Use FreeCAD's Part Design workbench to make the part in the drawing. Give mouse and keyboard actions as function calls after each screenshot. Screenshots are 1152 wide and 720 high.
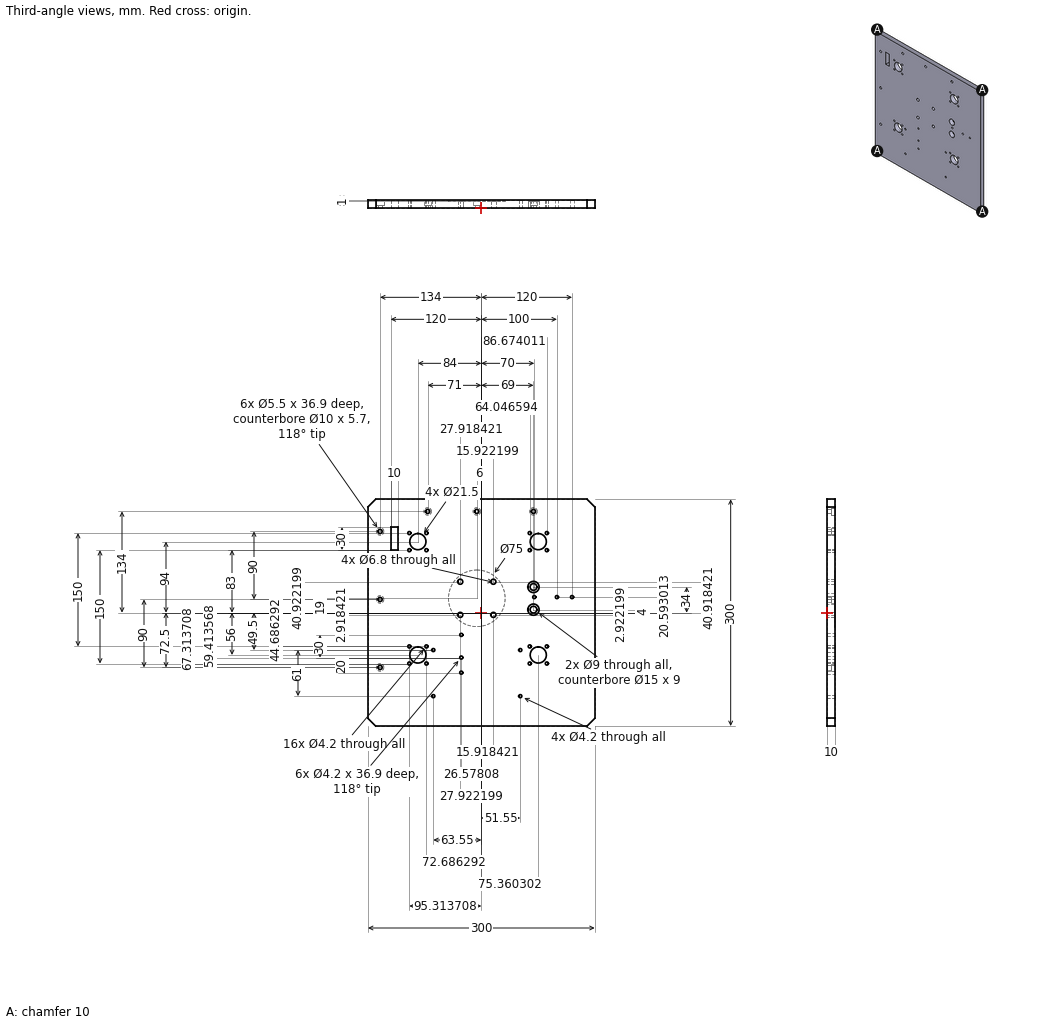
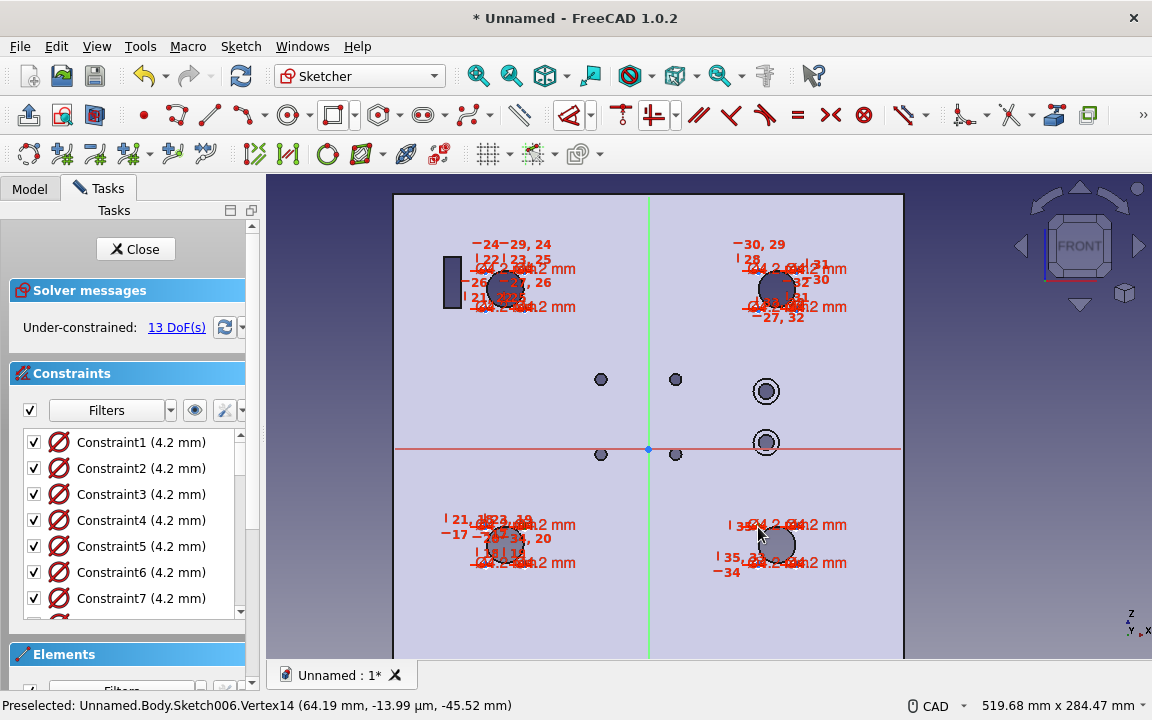
key(h)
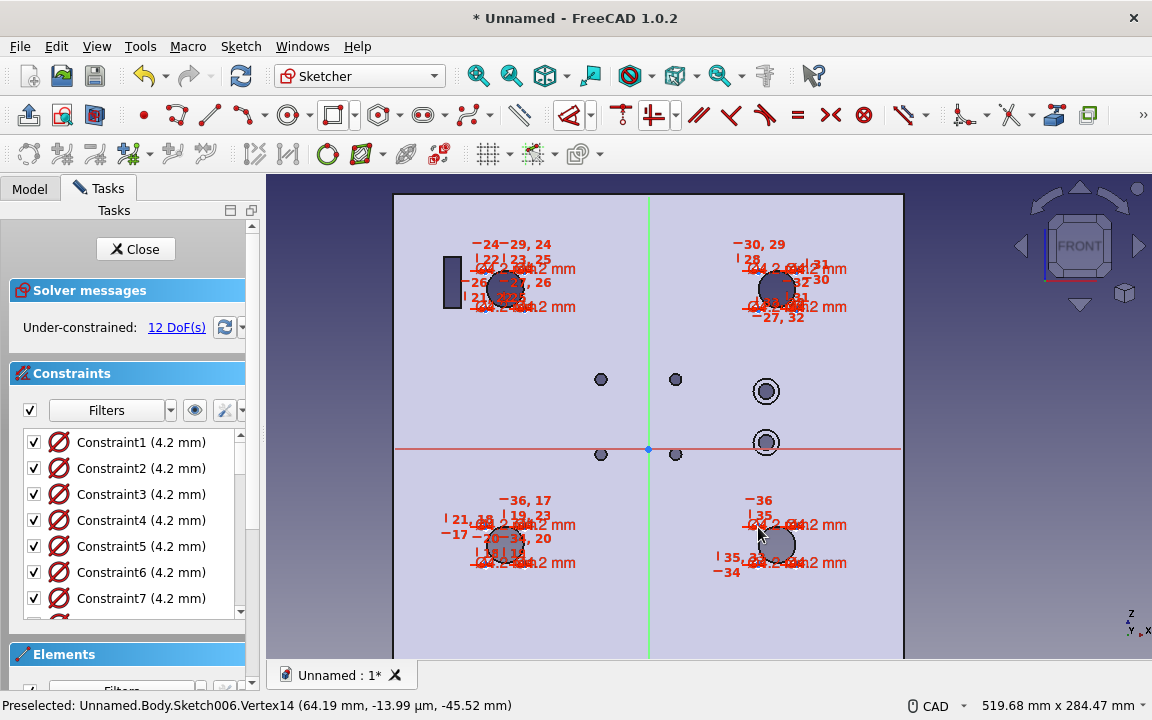
click(796, 309)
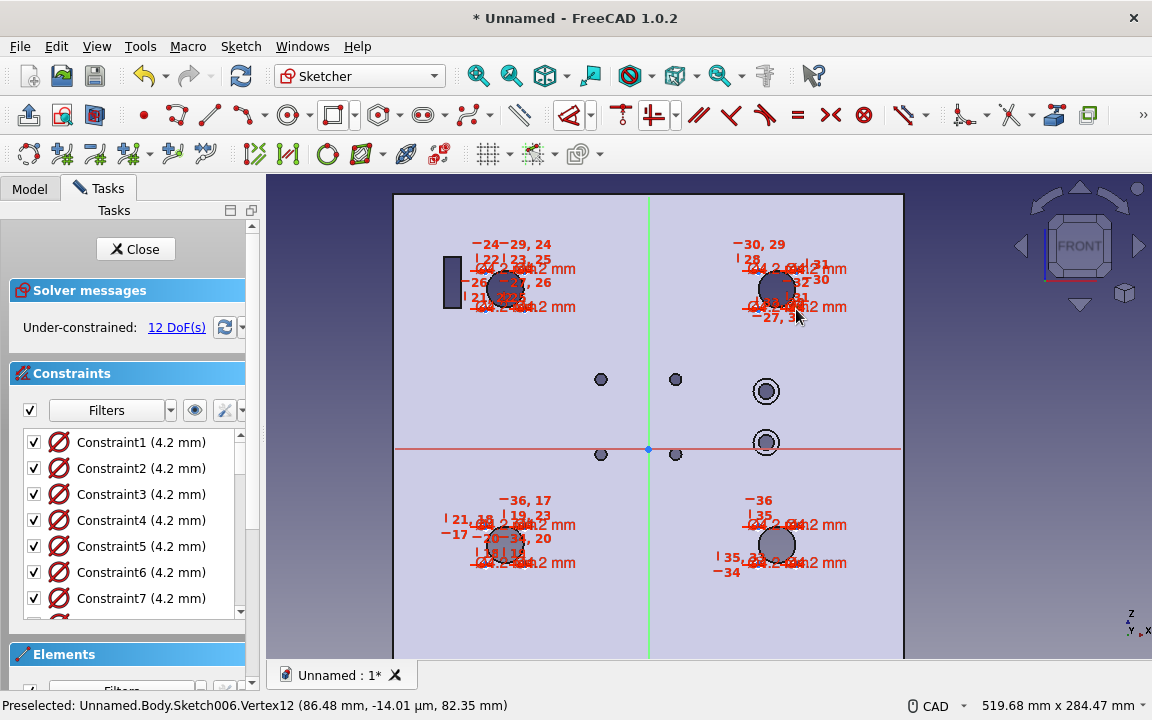
click(796, 527)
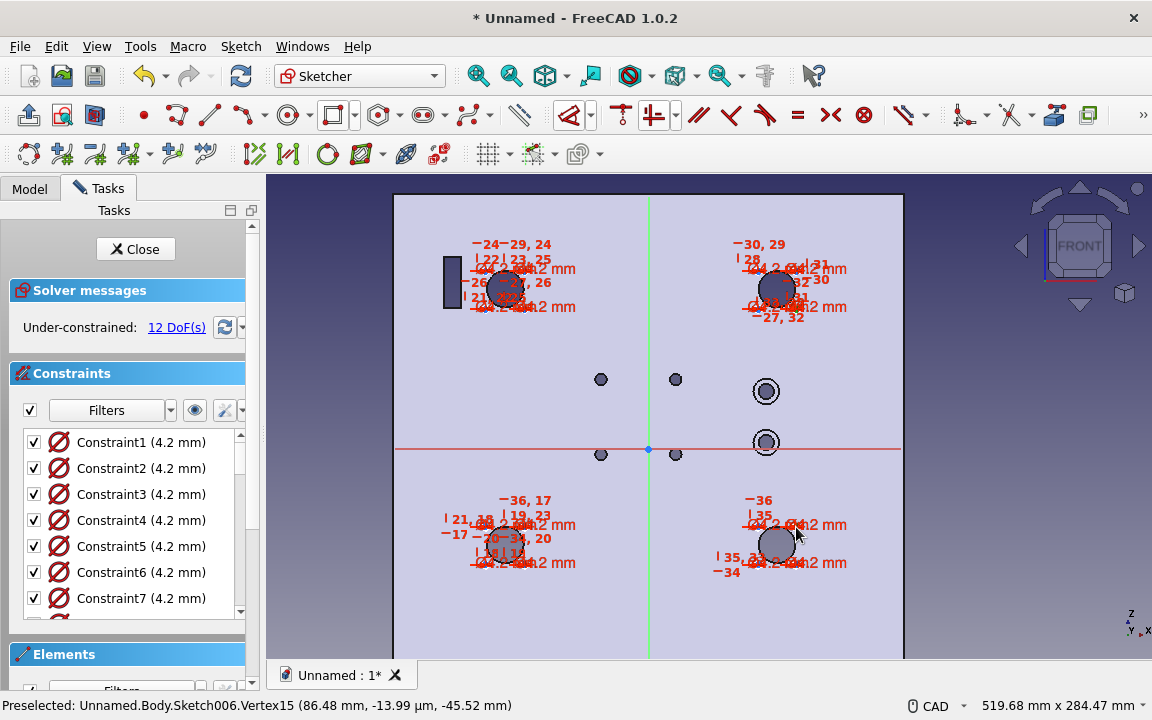
click(676, 116)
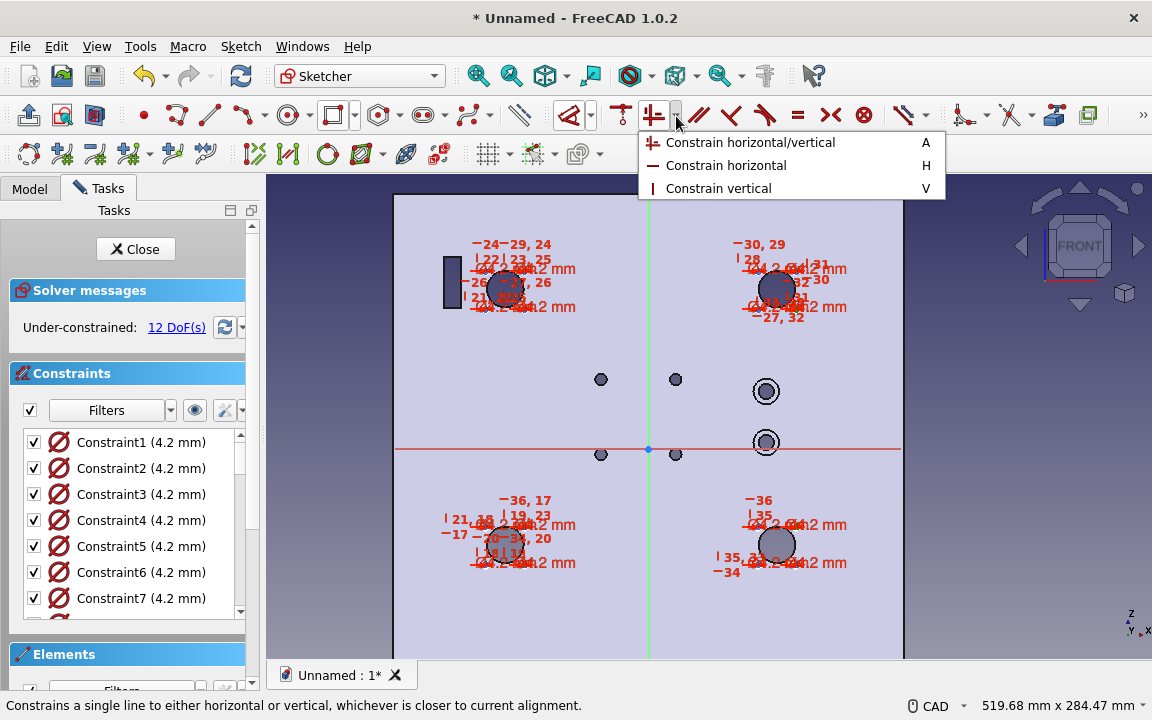
click(792, 188)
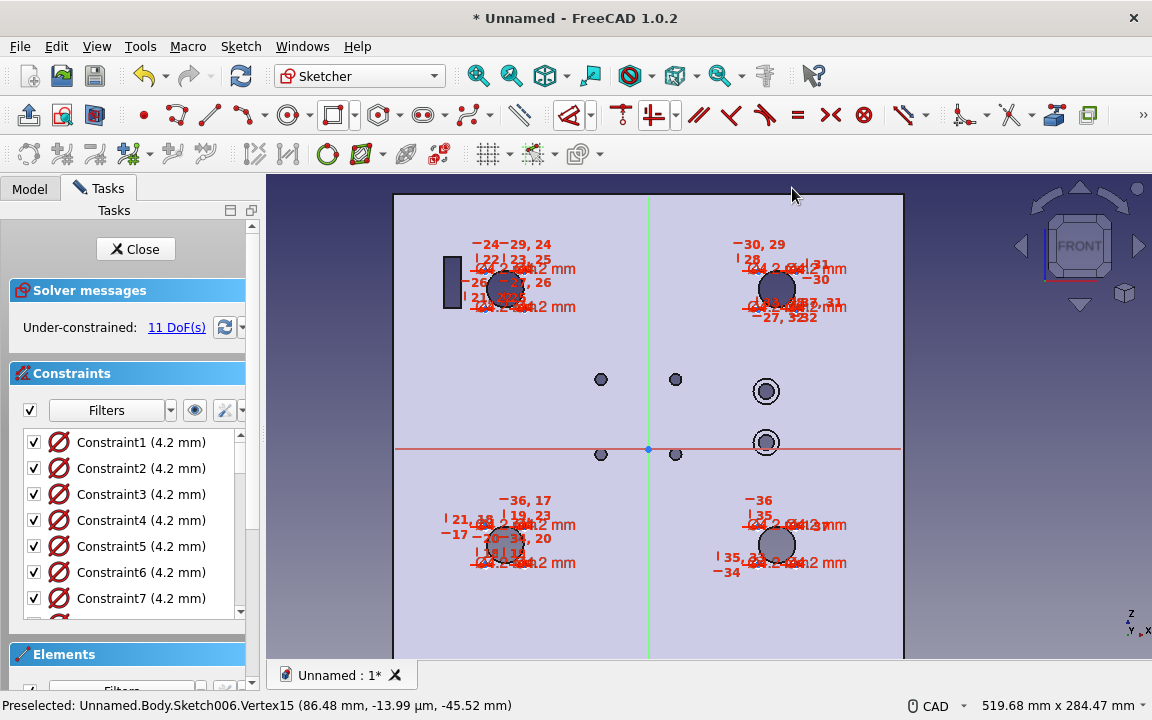
click(758, 527)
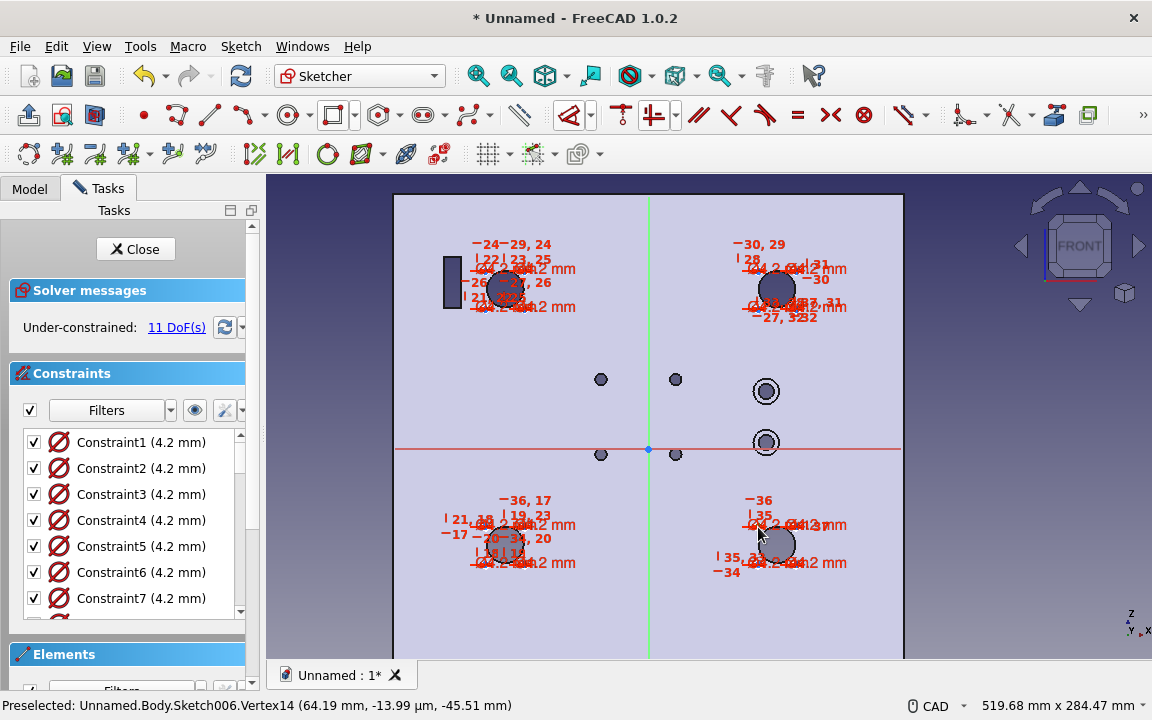
click(796, 527)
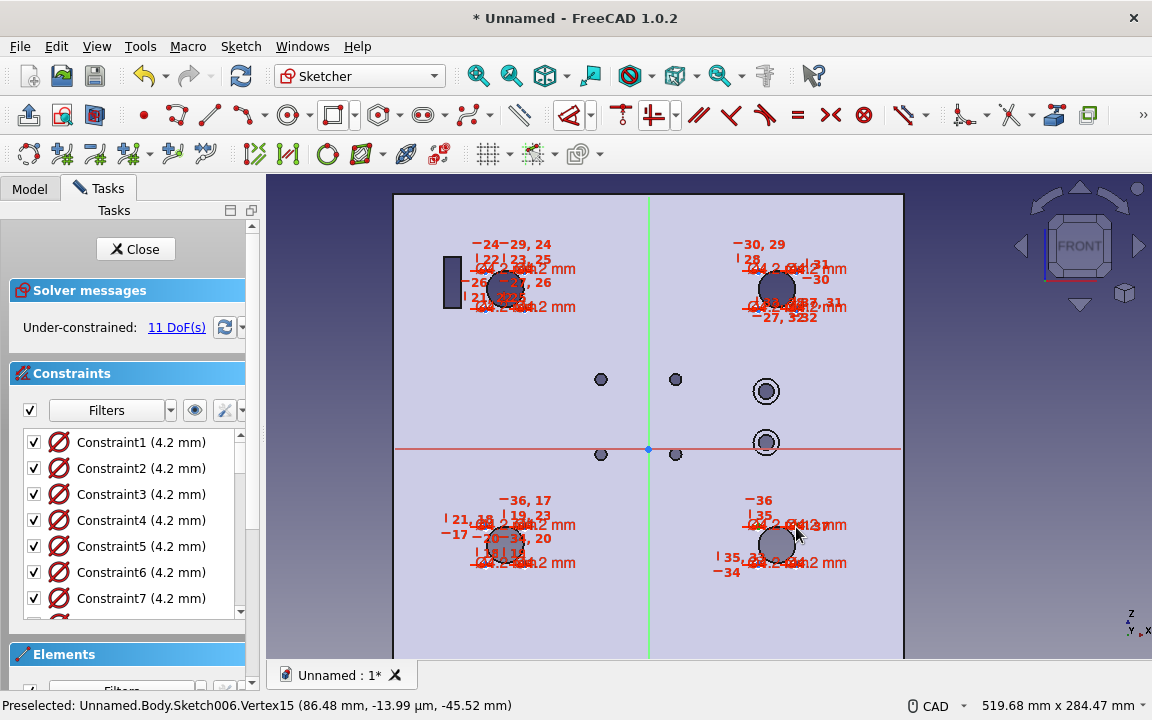
click(676, 116)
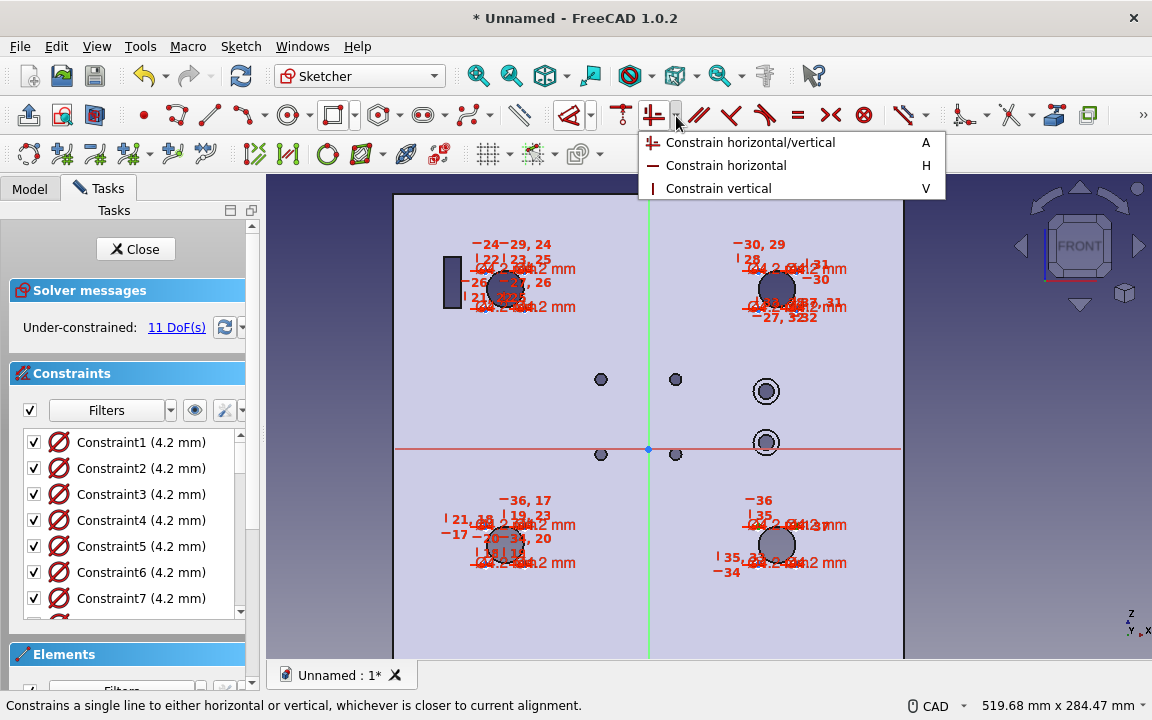
click(792, 166)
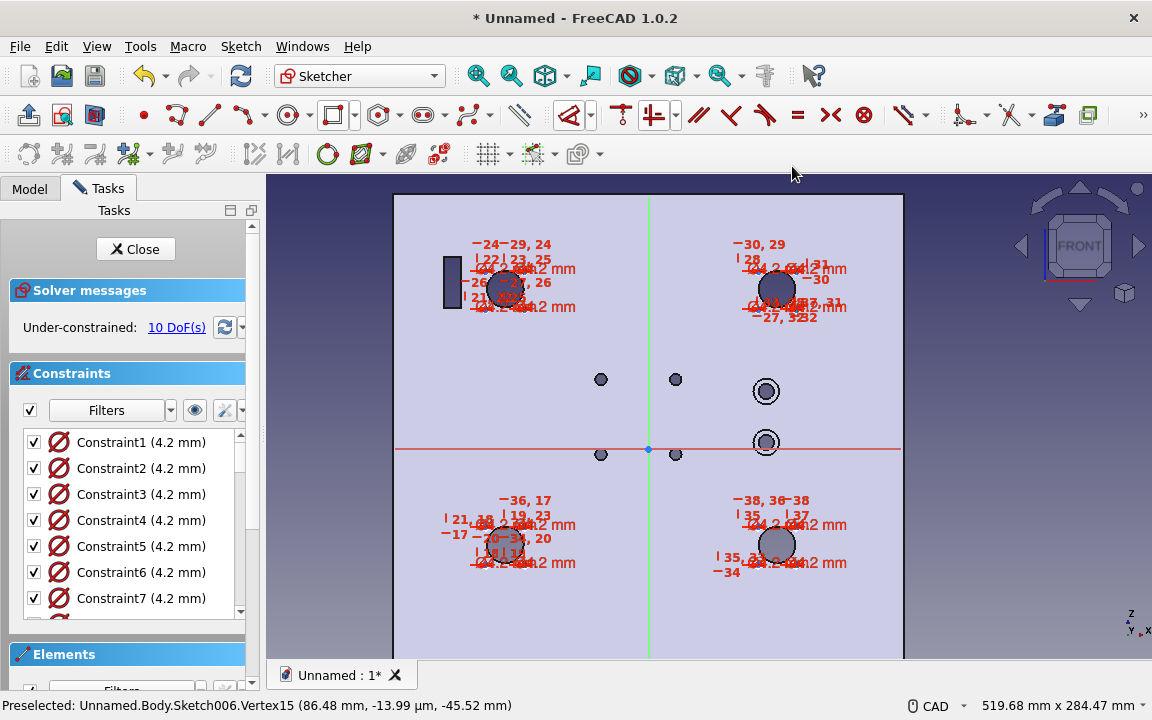
click(796, 527)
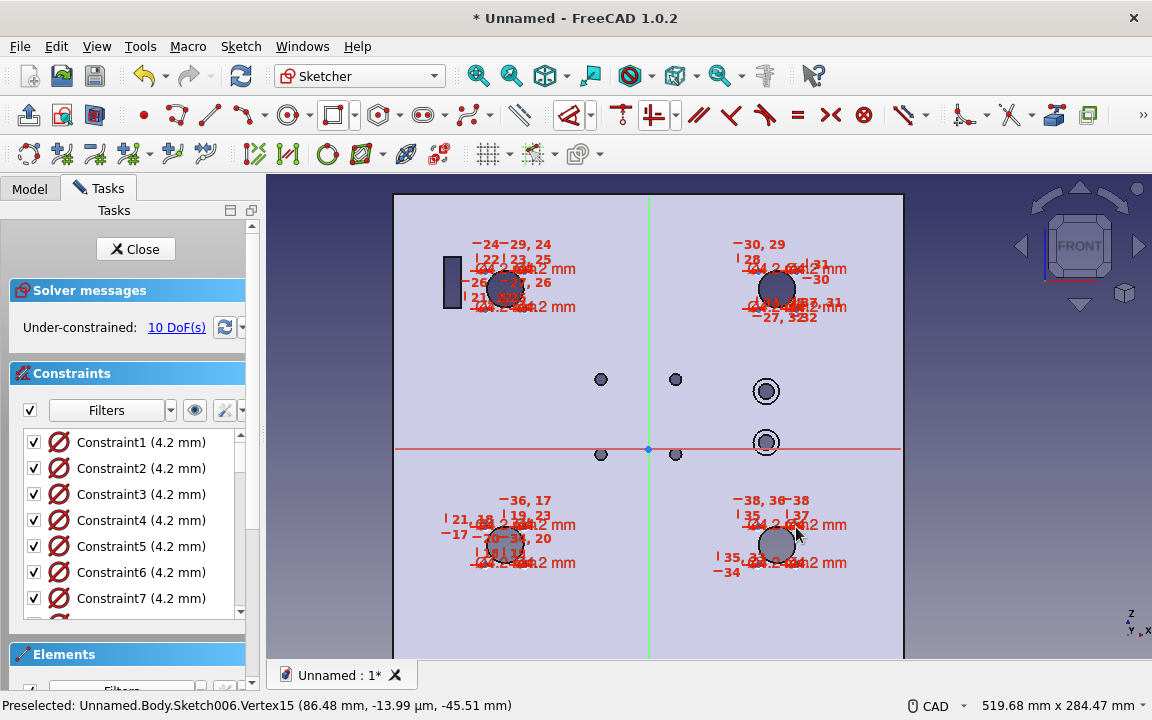
click(796, 565)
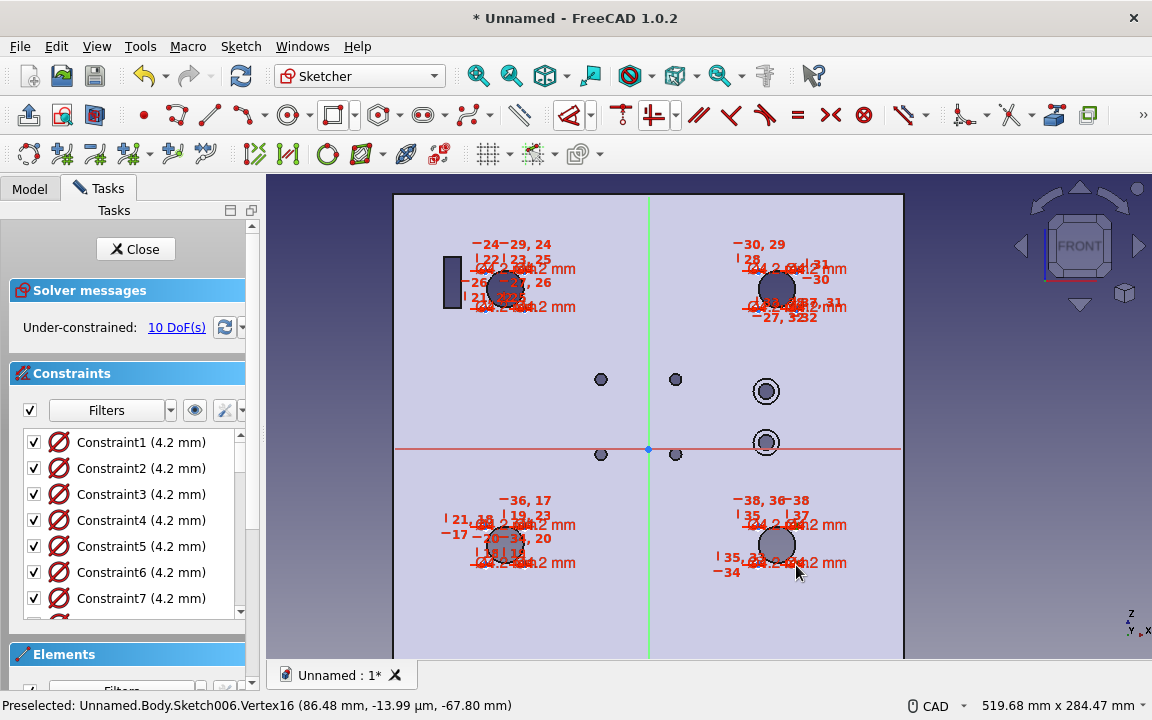
click(676, 116)